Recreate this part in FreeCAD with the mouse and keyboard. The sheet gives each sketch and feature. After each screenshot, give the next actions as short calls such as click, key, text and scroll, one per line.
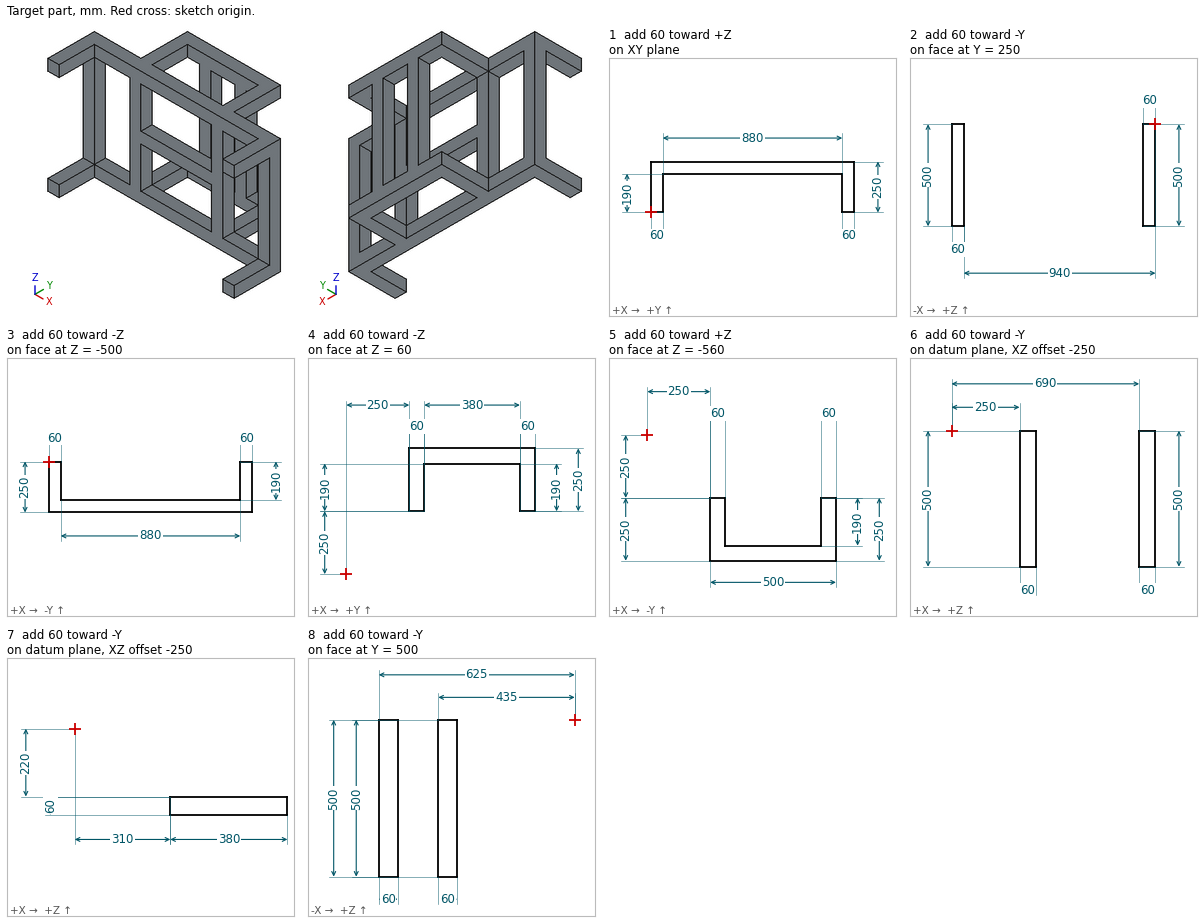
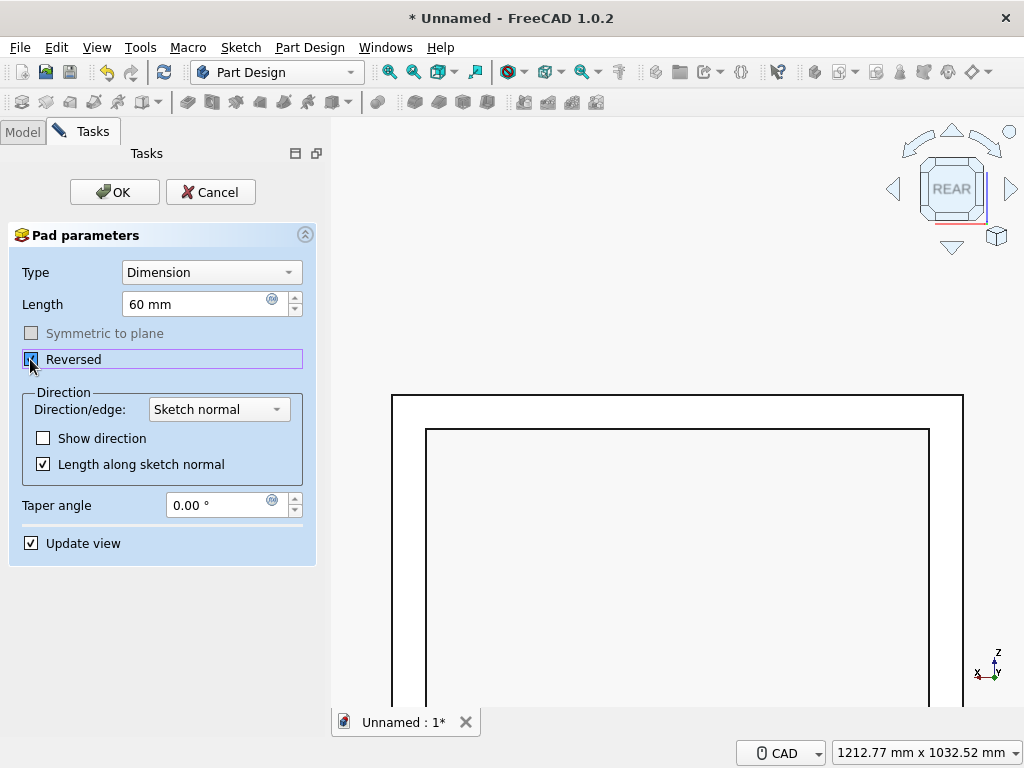
click(115, 192)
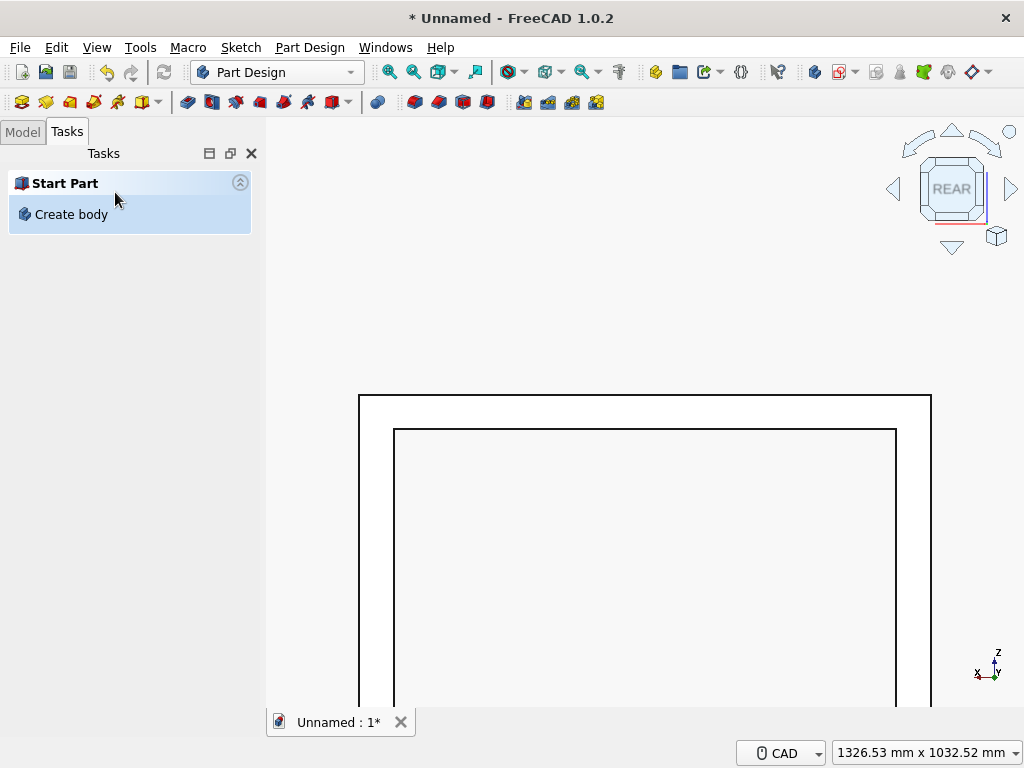
click(390, 72)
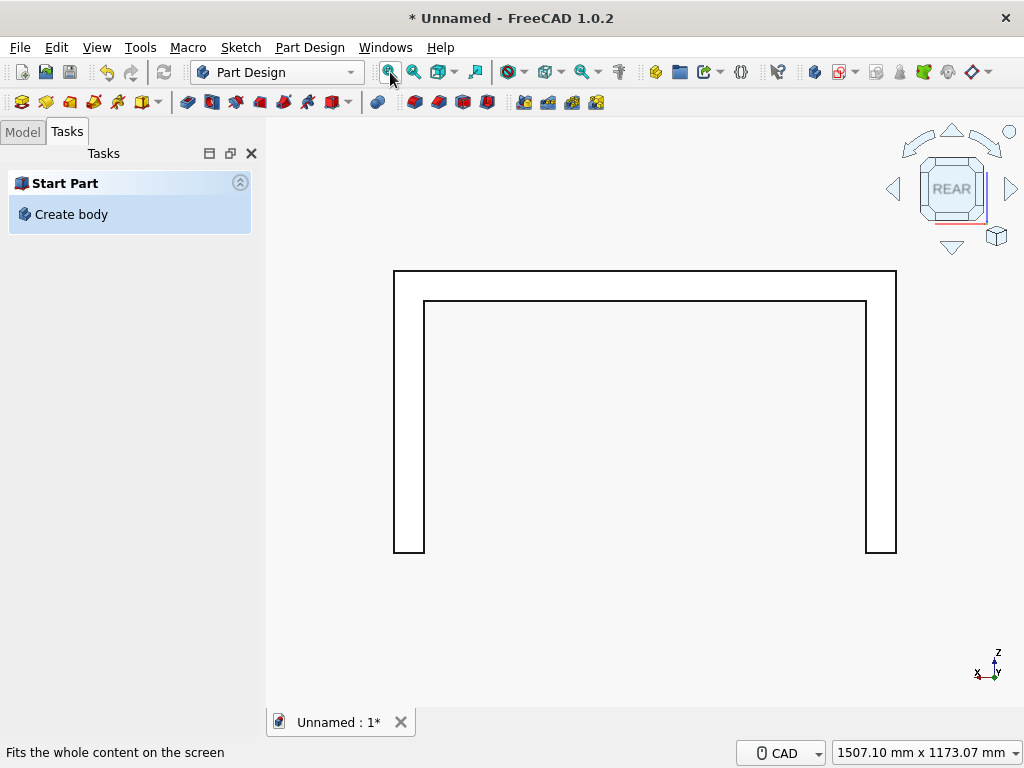
key(5)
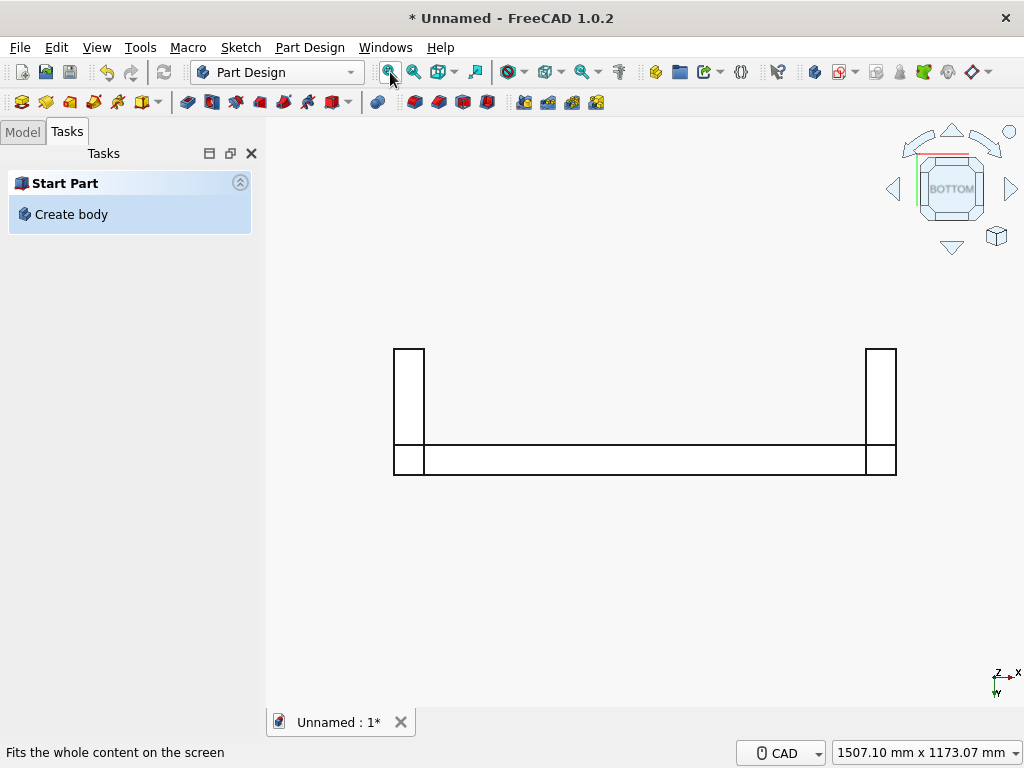
click(409, 459)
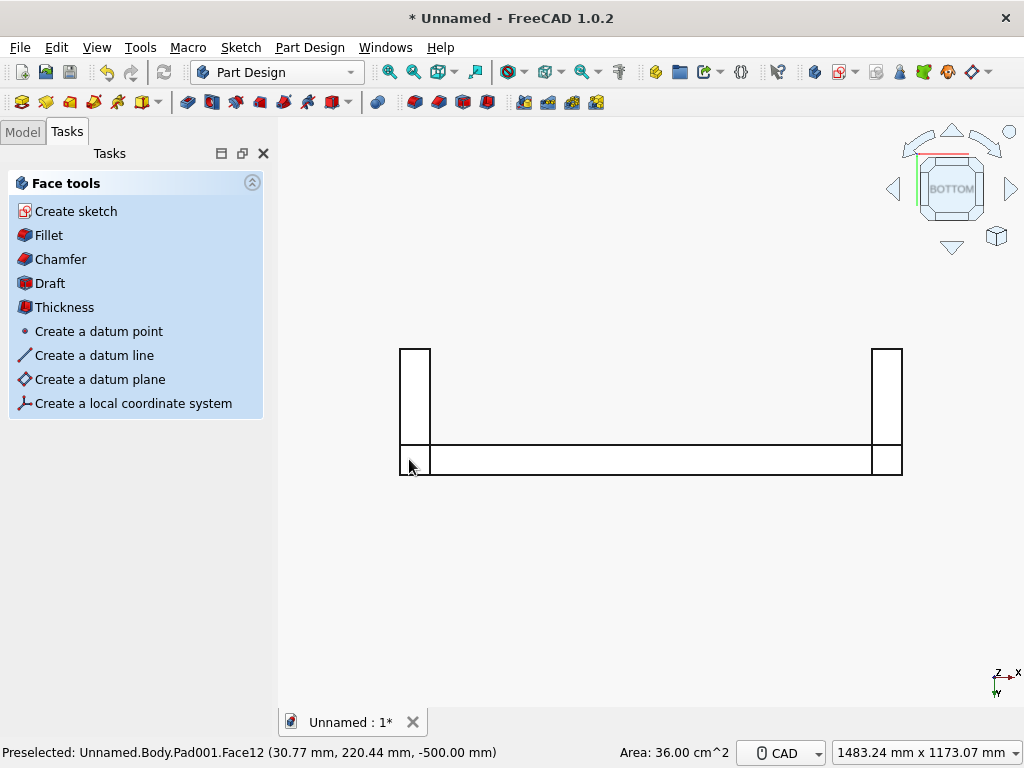
click(840, 72)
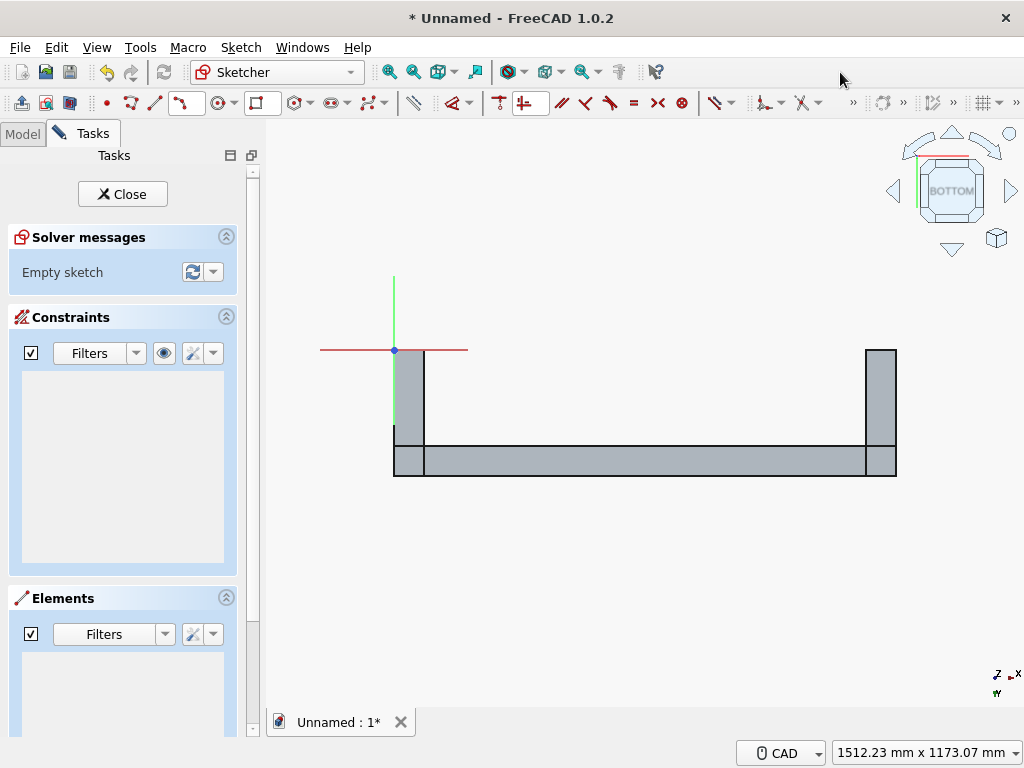
scroll(294, 413, down, 1)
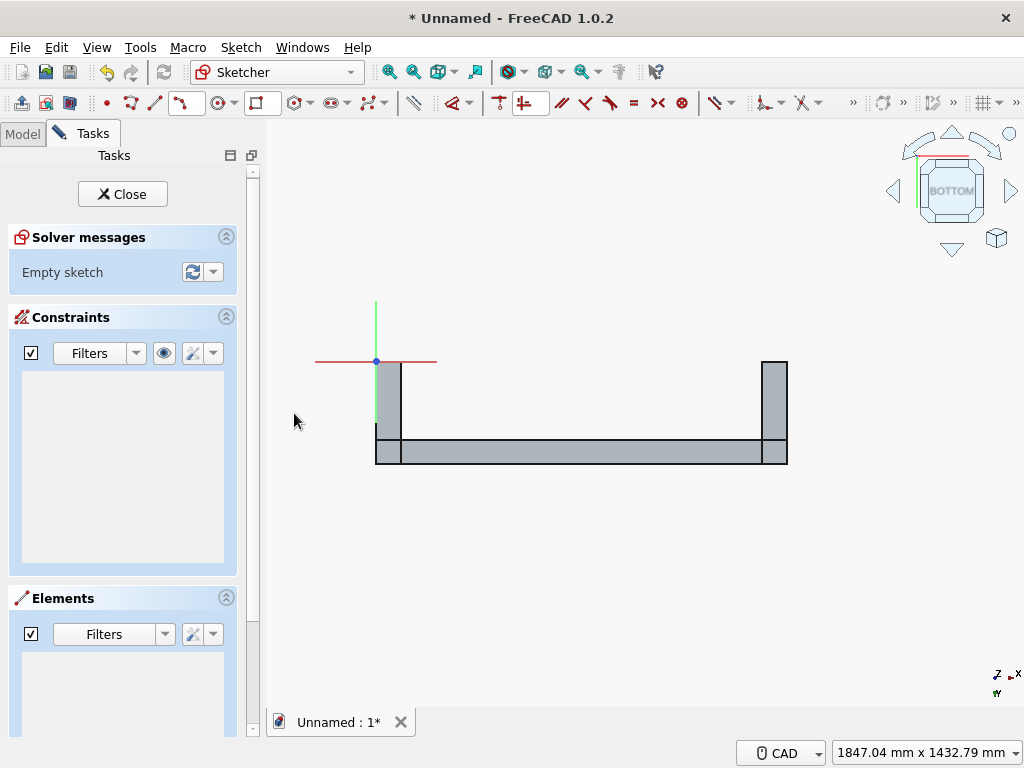
click(132, 104)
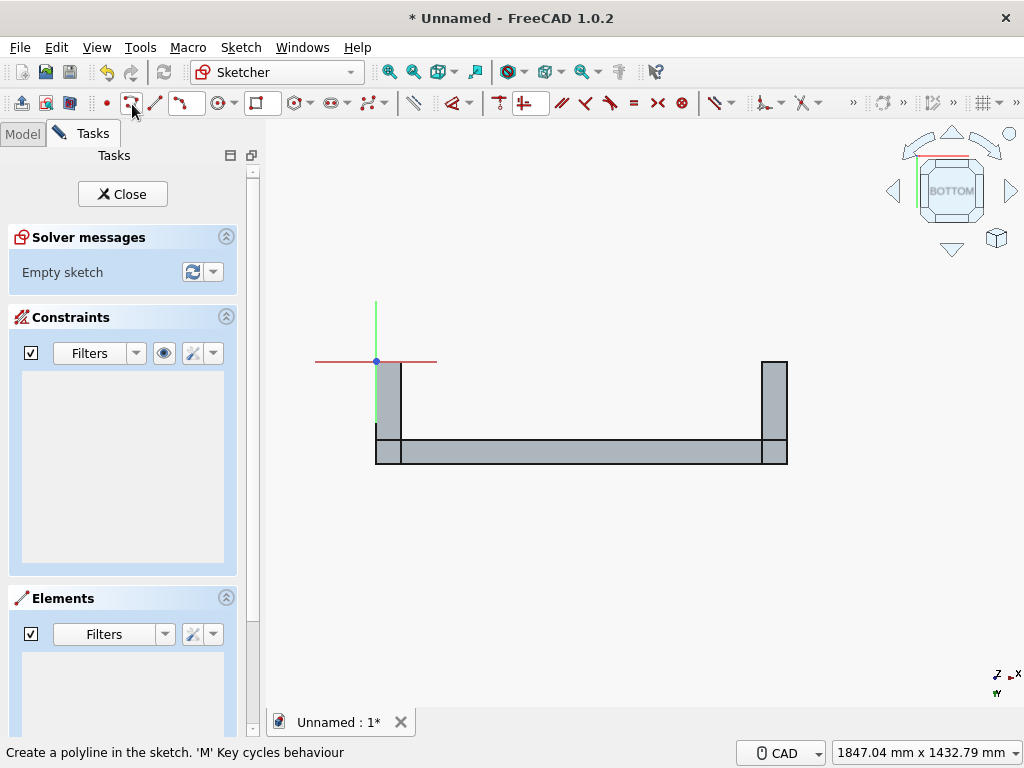
click(376, 362)
click(385, 464)
click(787, 464)
click(787, 362)
click(762, 371)
click(762, 440)
click(401, 440)
click(401, 371)
click(376, 362)
key(Escape)
key(Escape)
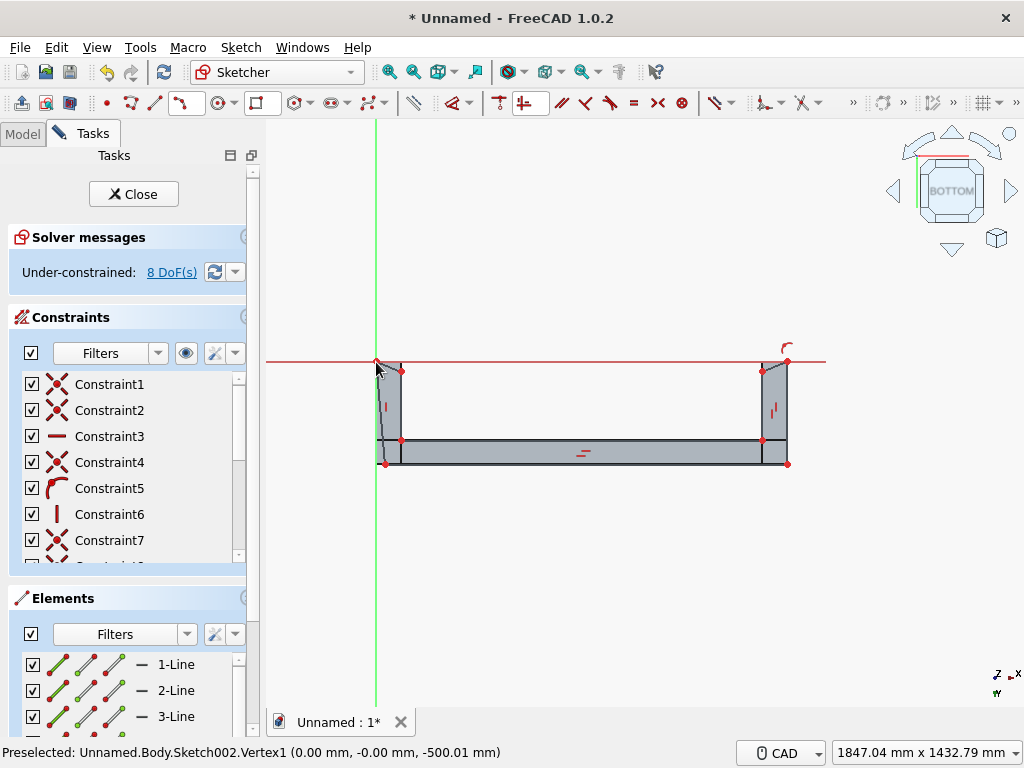
click(379, 393)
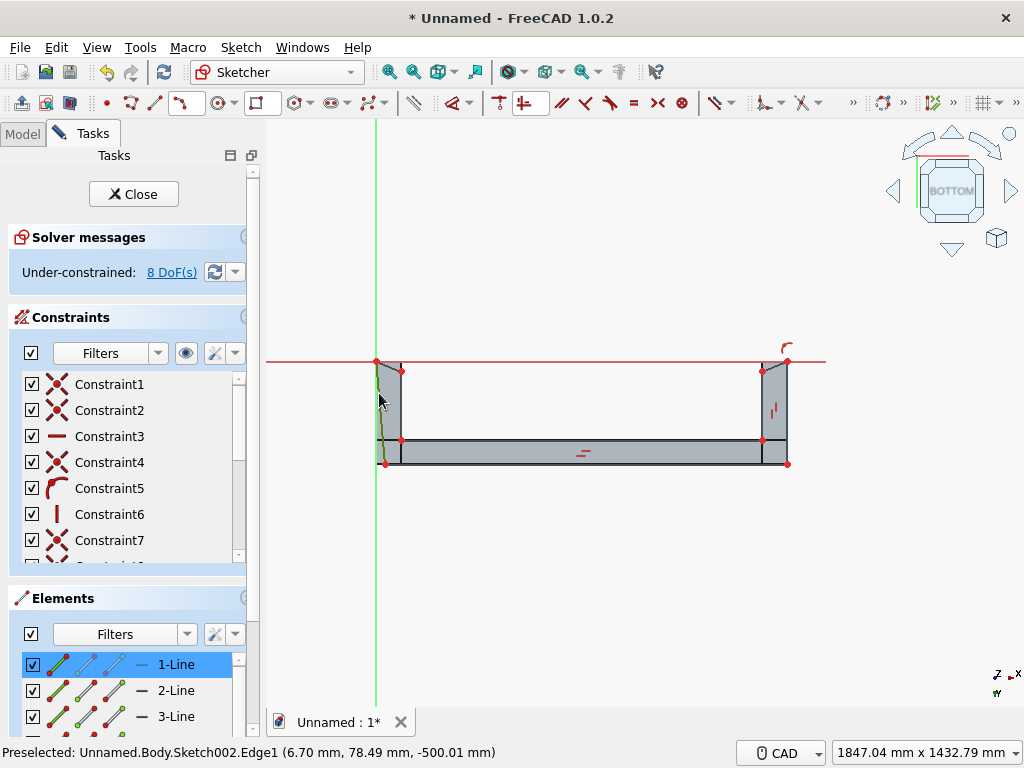
key(v)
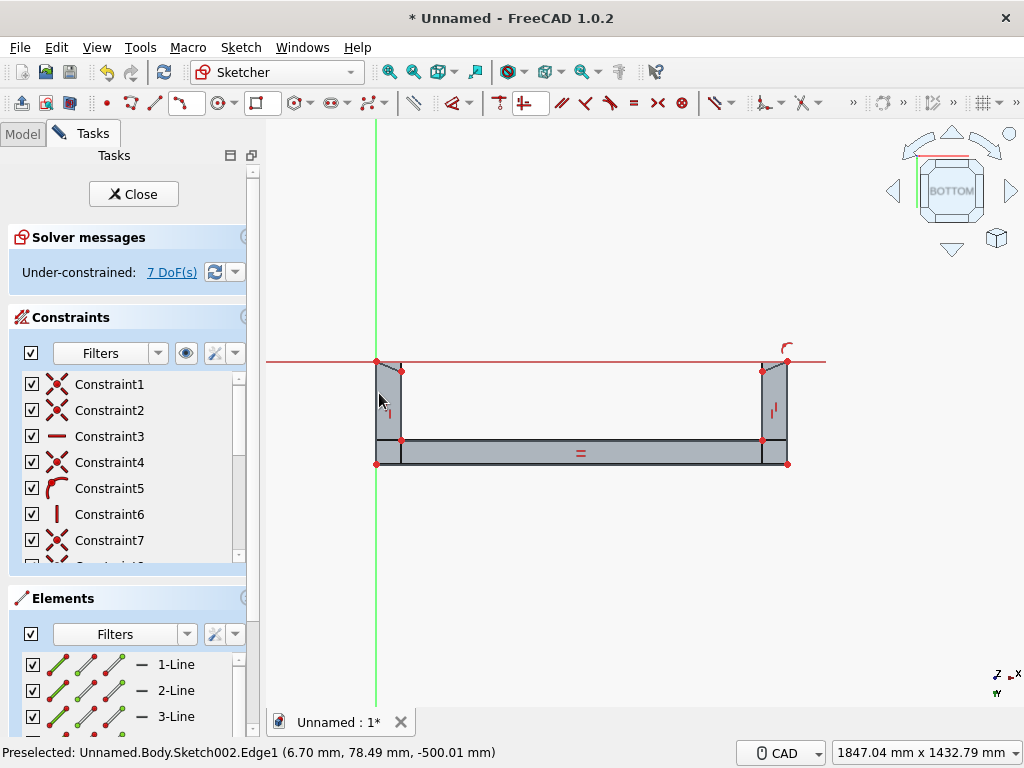
scroll(779, 365, up, 4)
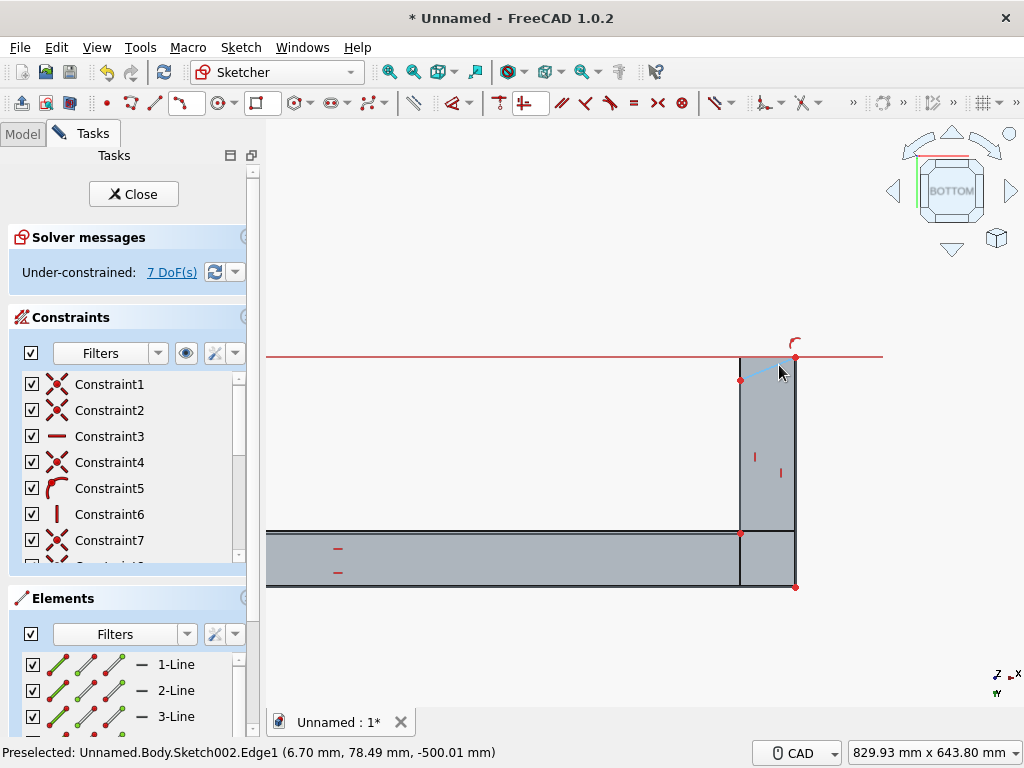
click(779, 364)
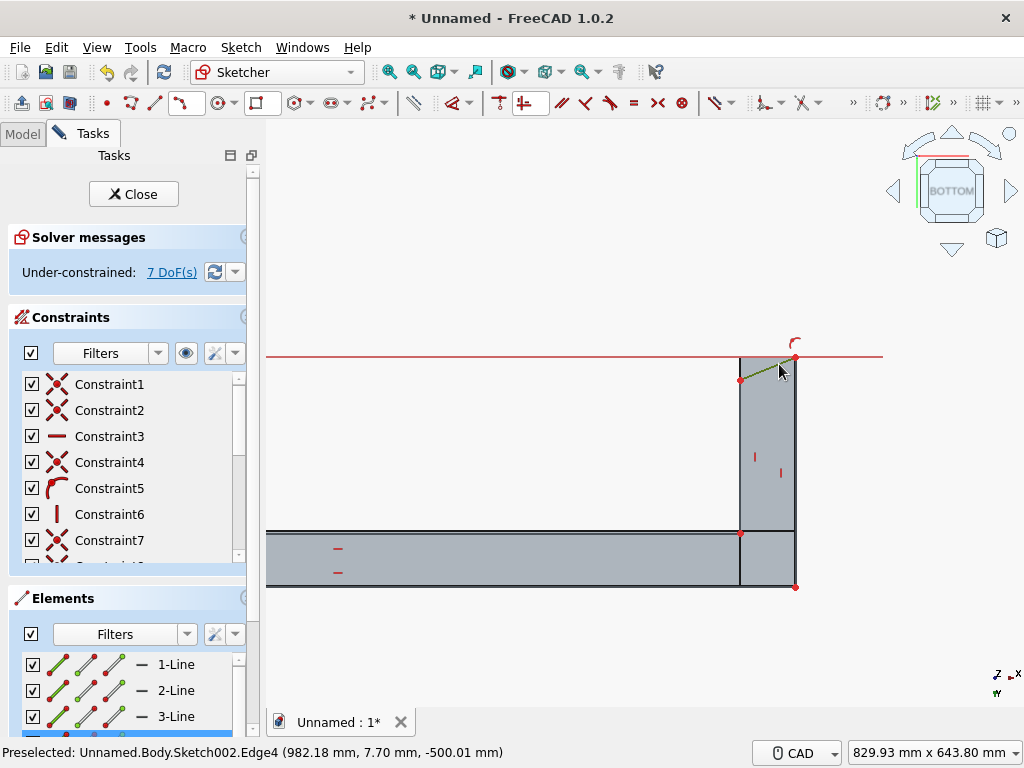
key(h)